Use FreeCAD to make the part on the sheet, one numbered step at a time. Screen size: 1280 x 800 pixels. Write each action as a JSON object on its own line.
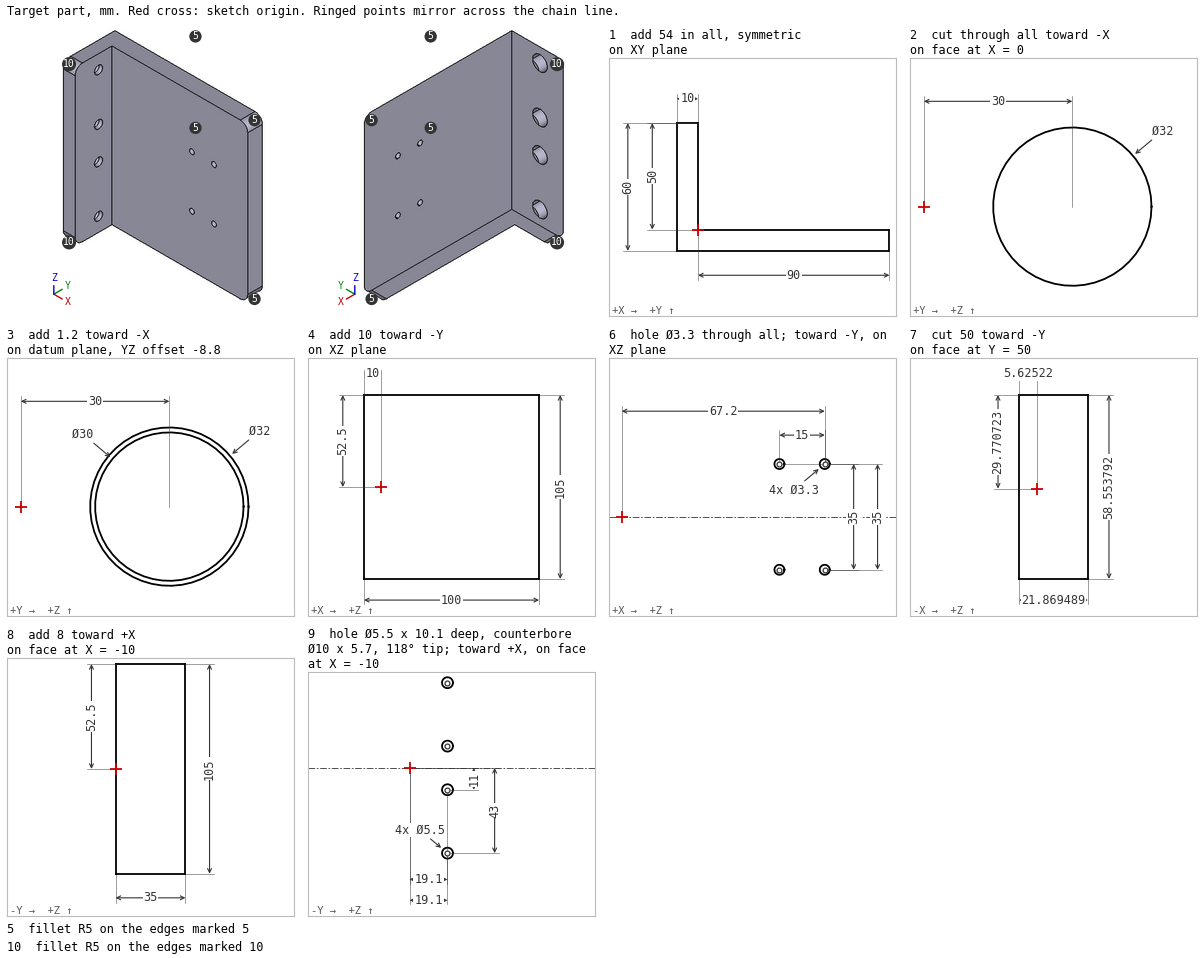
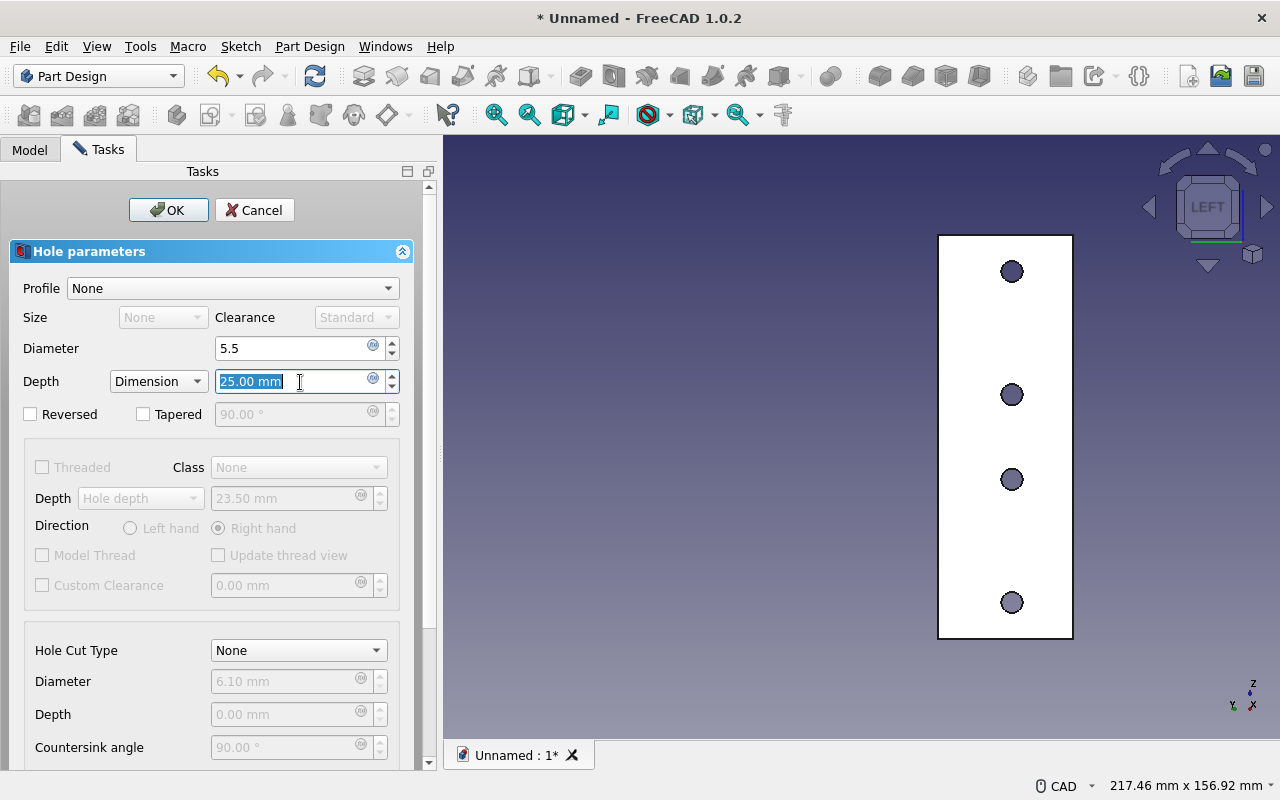
{"action": "type", "text": "10.1"}
{"action": "key", "text": "Tab"}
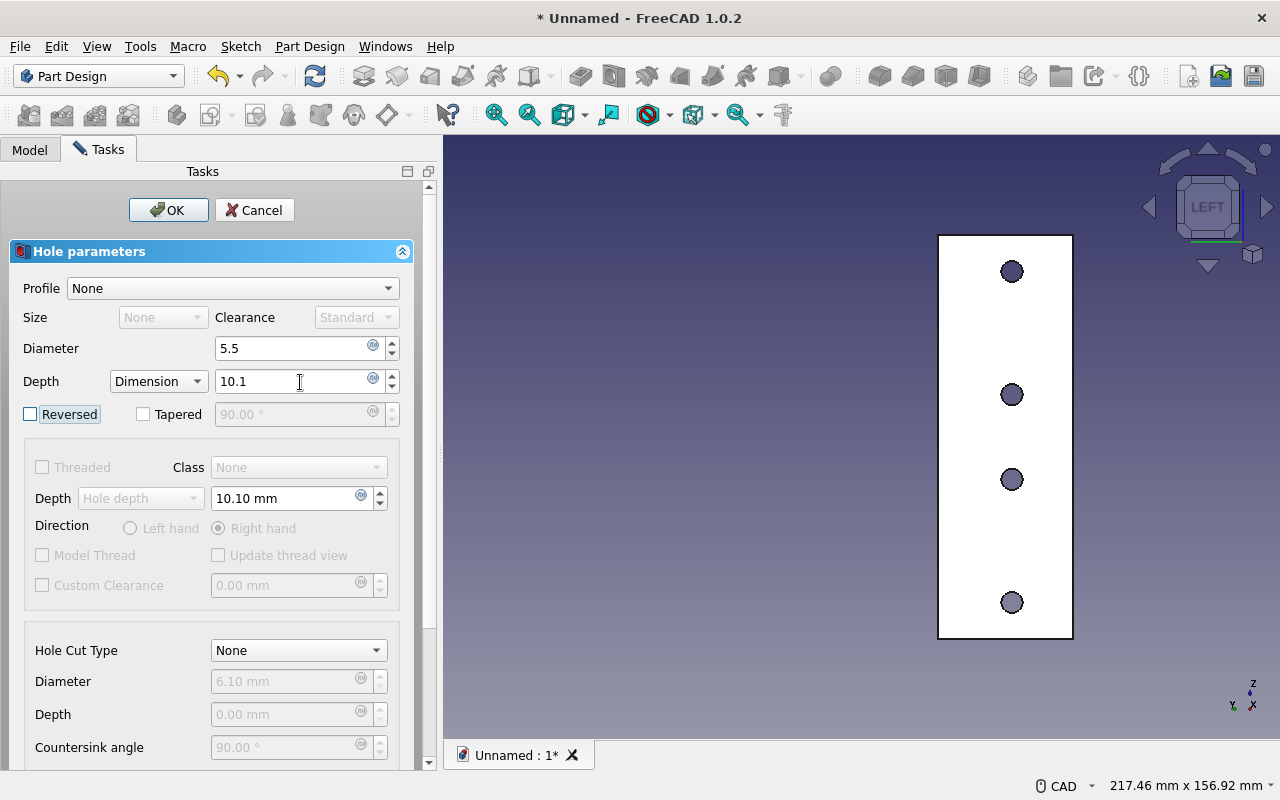
{"action": "left_click", "coordinate": [300, 650]}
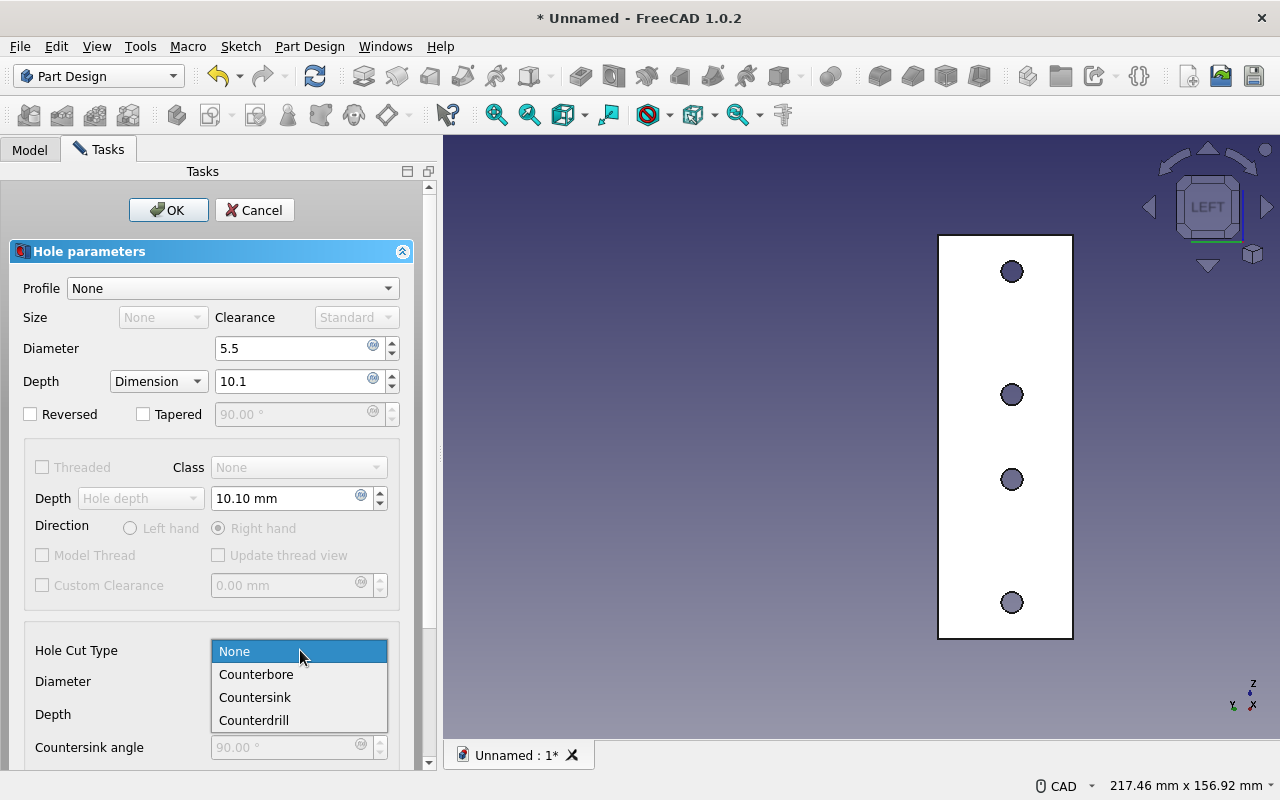
{"action": "left_click", "coordinate": [298, 674]}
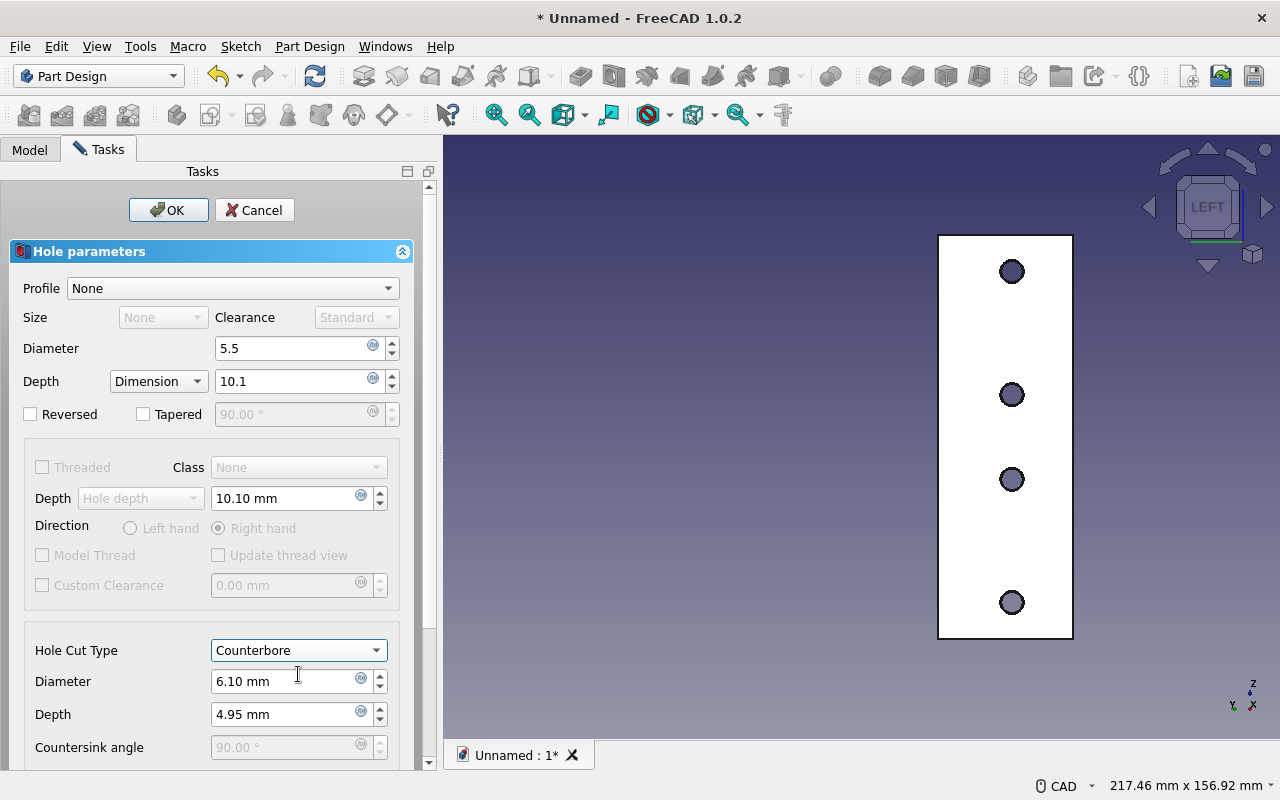
{"action": "triple_click", "coordinate": [292, 682]}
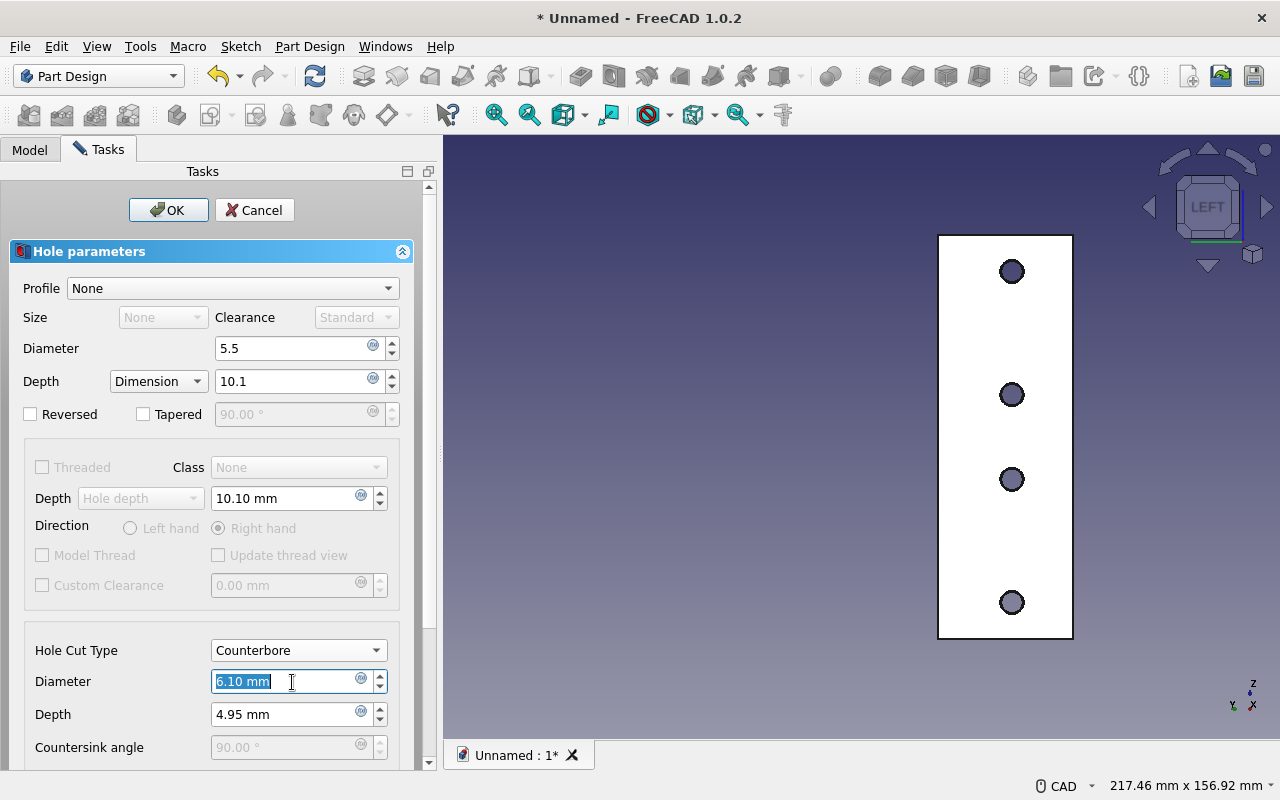
{"action": "type", "text": "10"}
{"action": "key", "text": "Tab"}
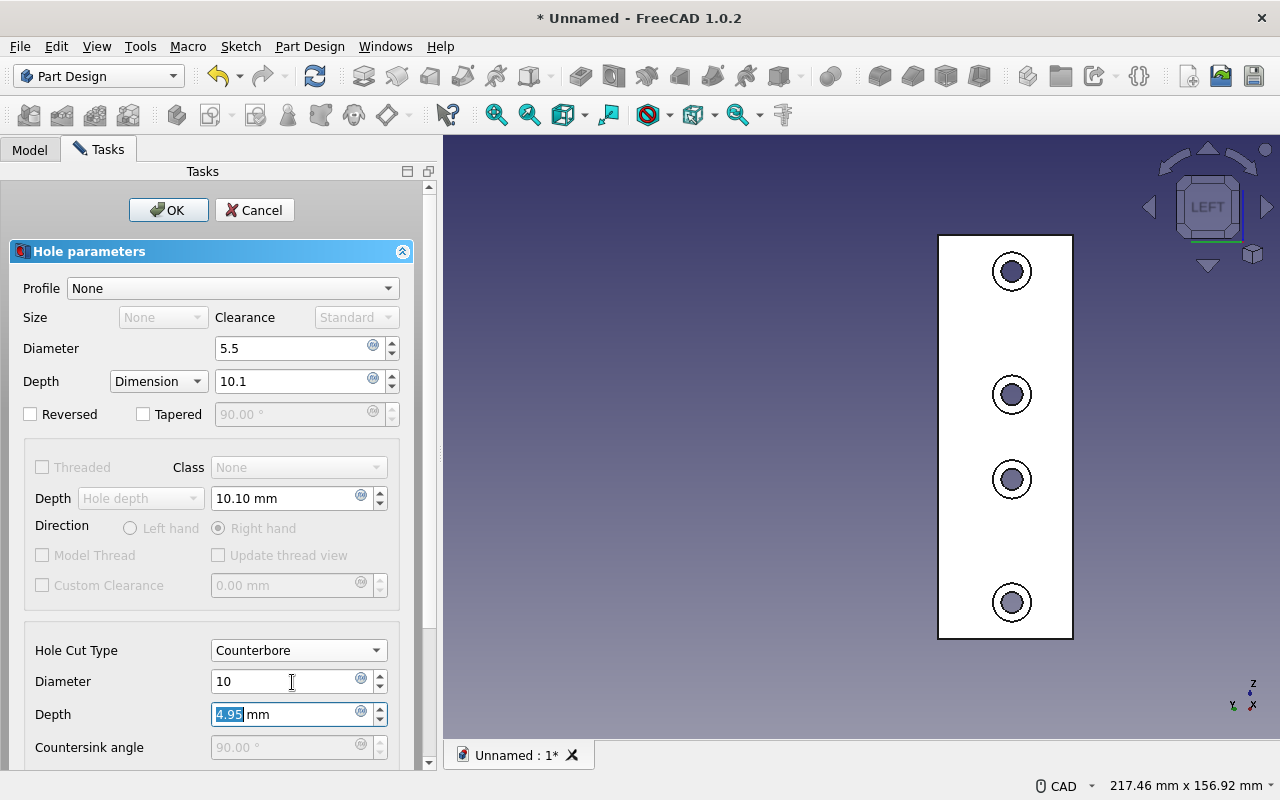
{"action": "type", "text": "5.7"}
{"action": "key", "text": "Tab"}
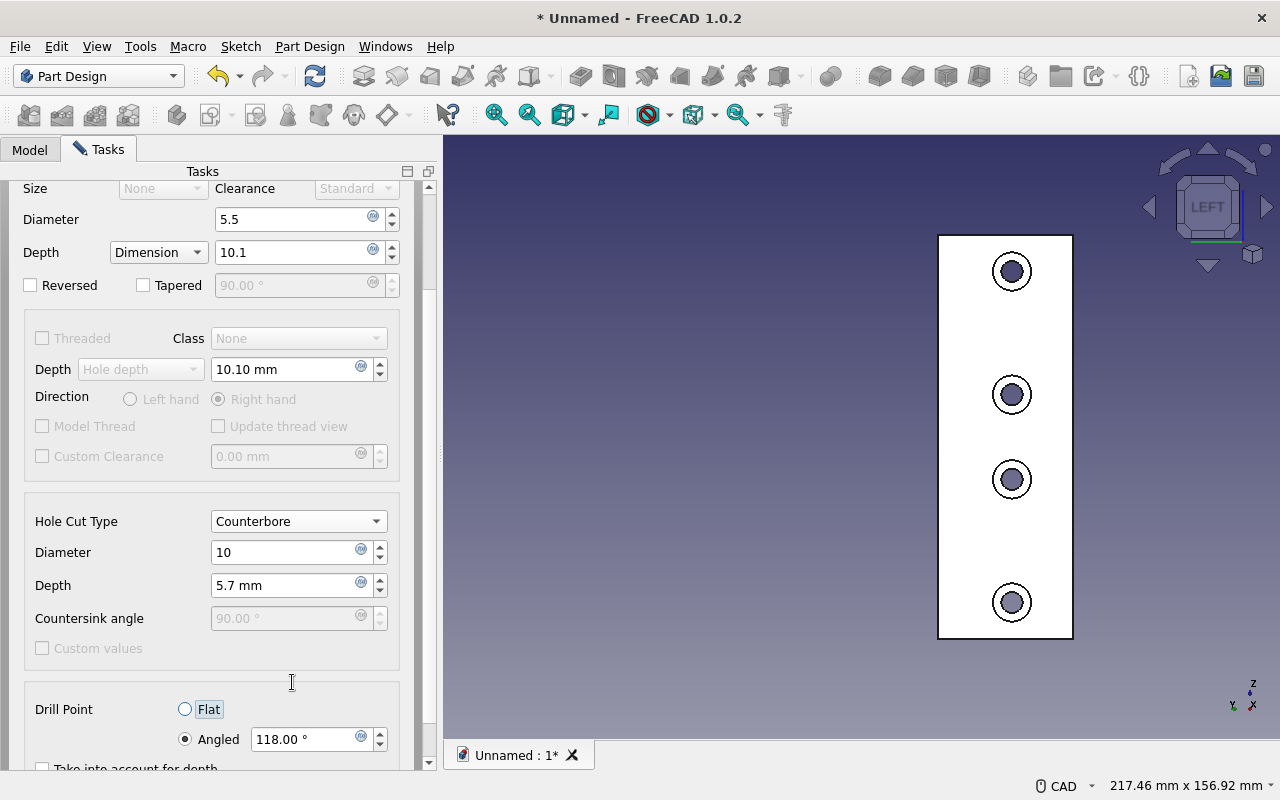
{"action": "scroll", "coordinate": [429, 476], "scroll_direction": "up", "scroll_amount": 3}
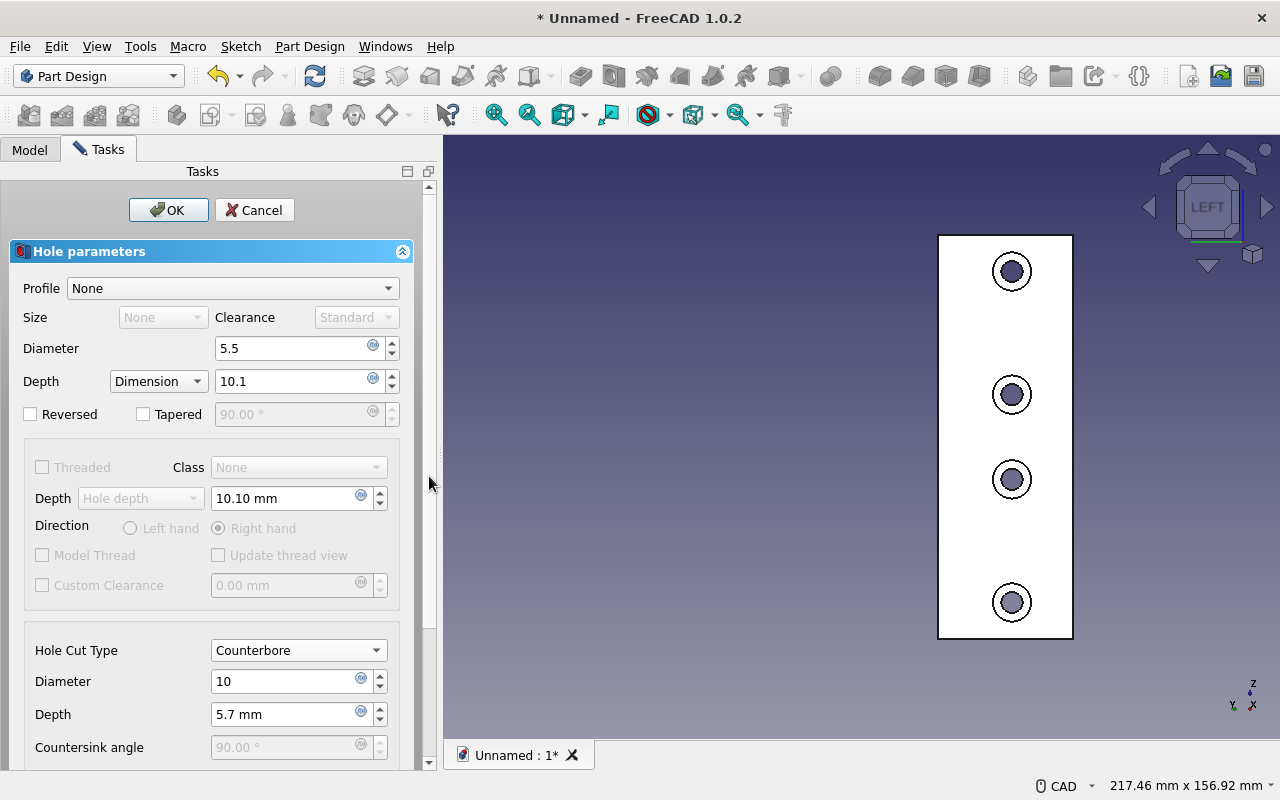
{"action": "left_click", "coordinate": [169, 210]}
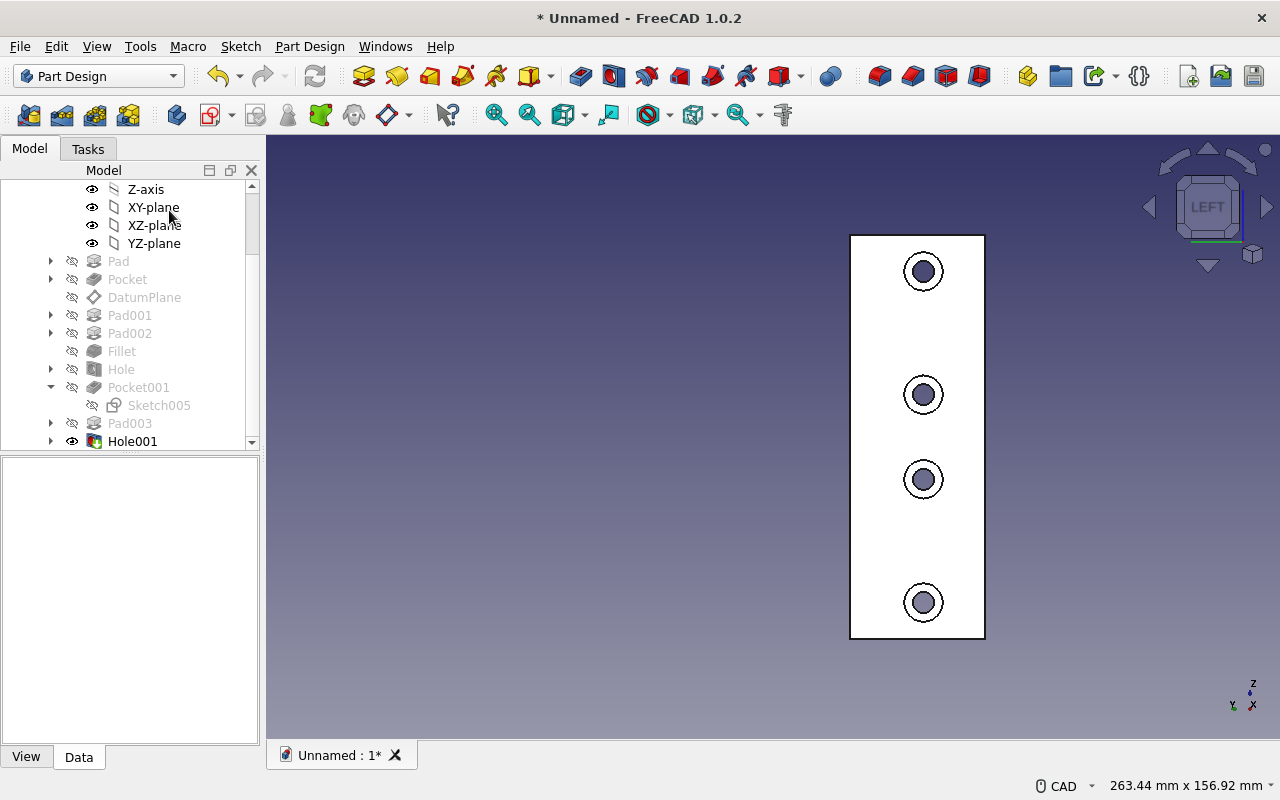
{"action": "key", "text": "0"}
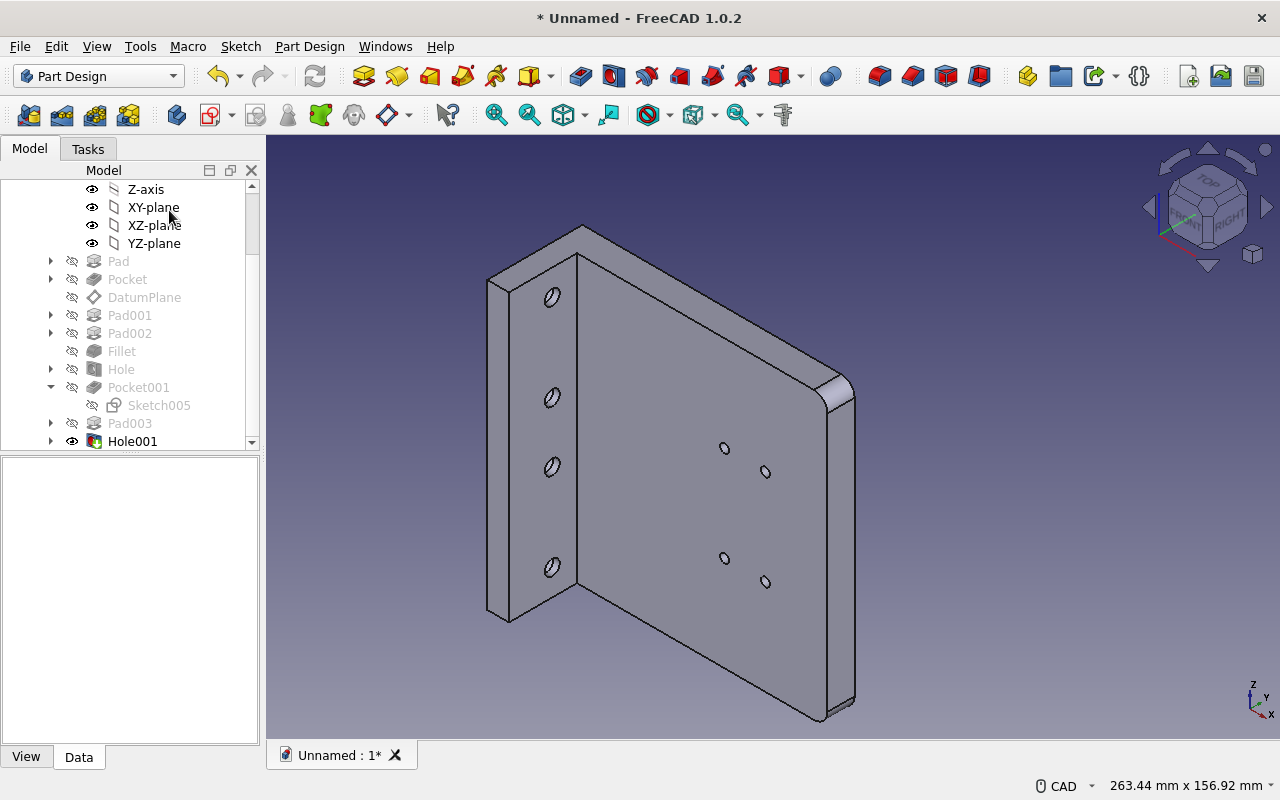
{"action": "left_click", "coordinate": [497, 116]}